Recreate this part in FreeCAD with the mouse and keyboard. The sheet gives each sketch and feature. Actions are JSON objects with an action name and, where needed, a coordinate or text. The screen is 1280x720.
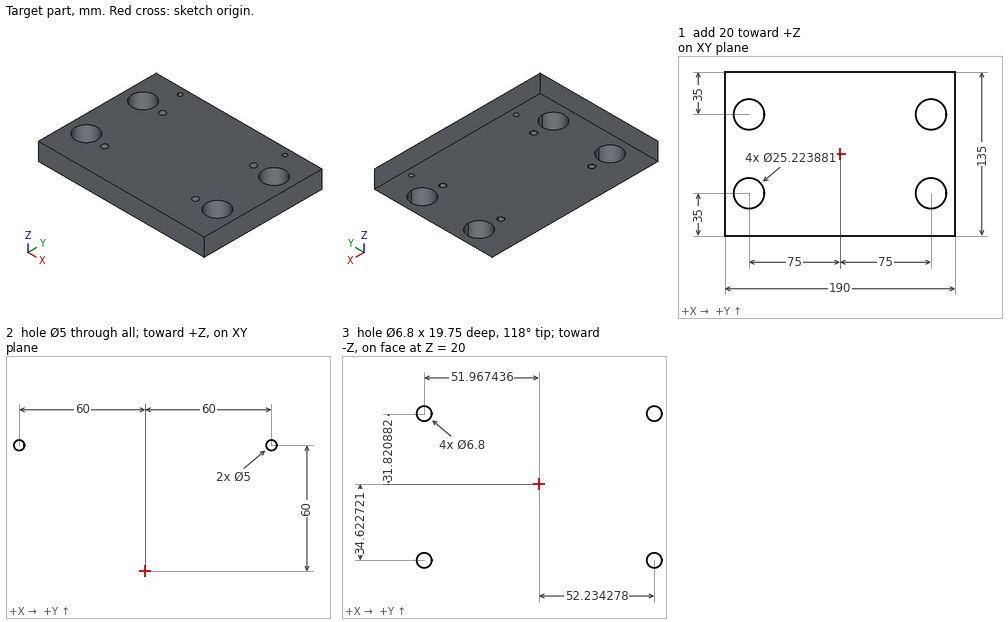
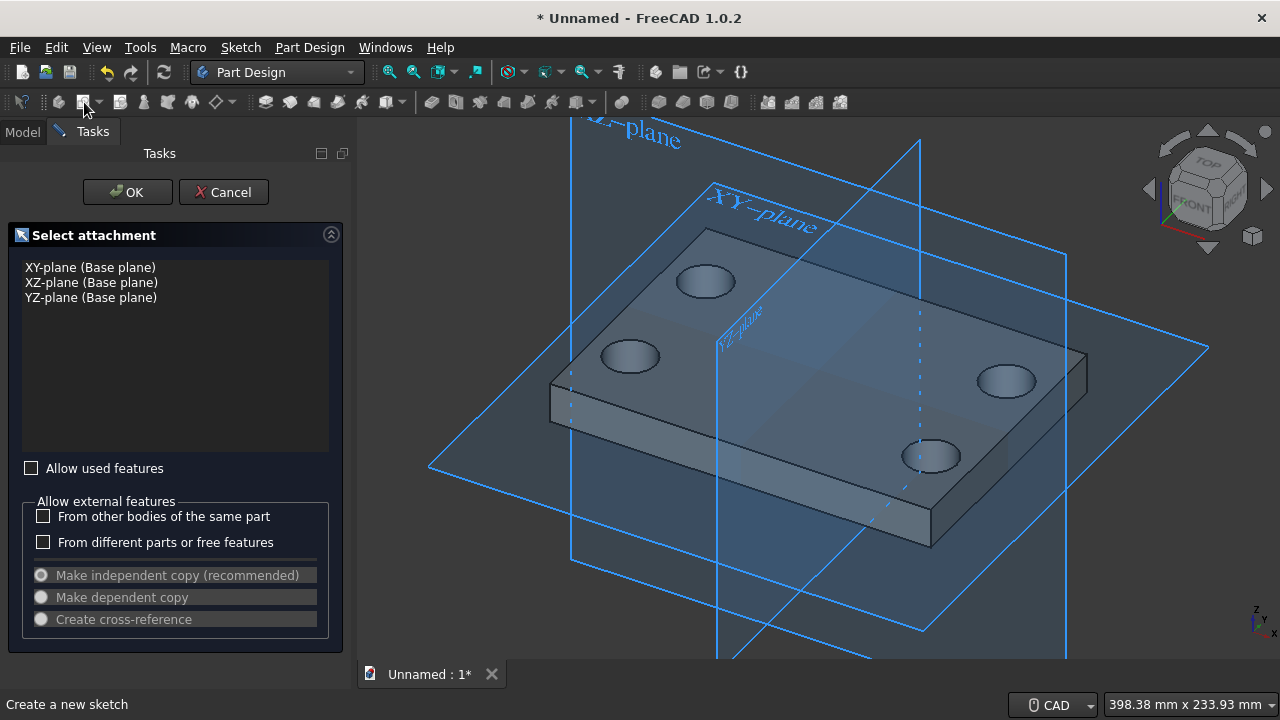
{"action": "left_click", "coordinate": [82, 268]}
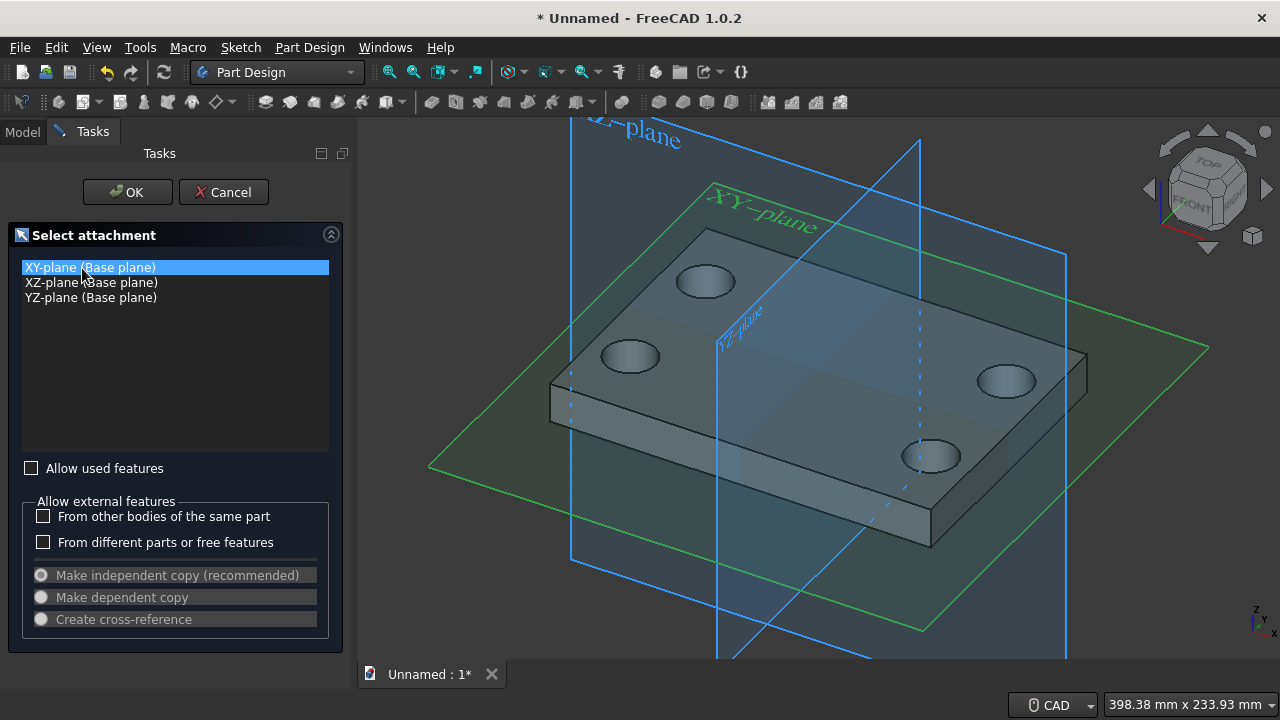
{"action": "left_click", "coordinate": [128, 192]}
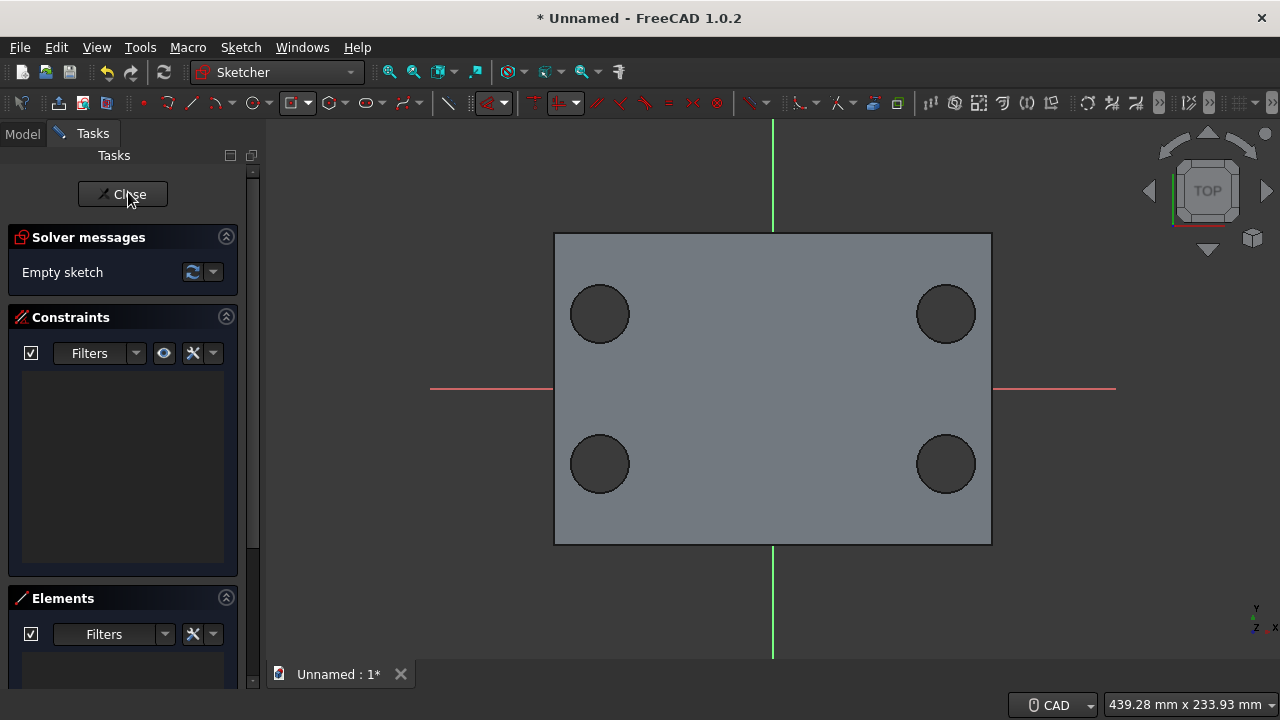
{"action": "left_click", "coordinate": [108, 104]}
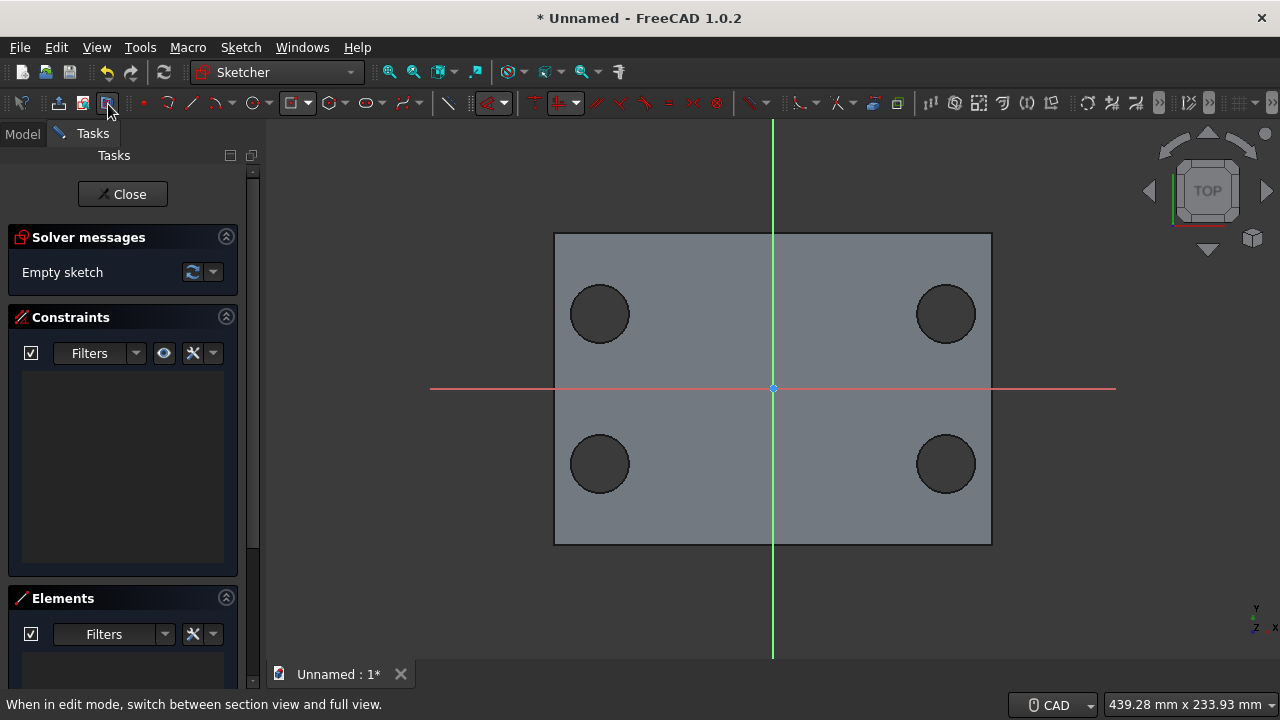
{"action": "scroll", "coordinate": [856, 229], "scroll_direction": "up", "scroll_amount": 3}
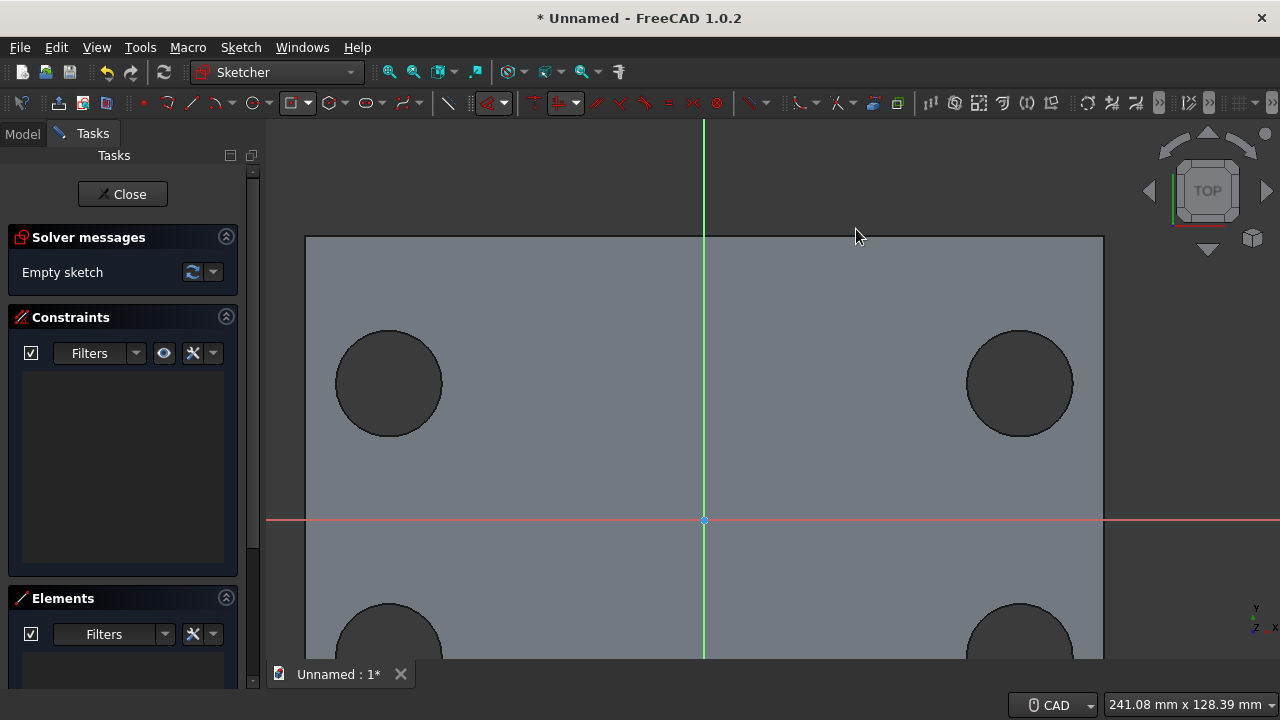
{"action": "key", "text": "g c"}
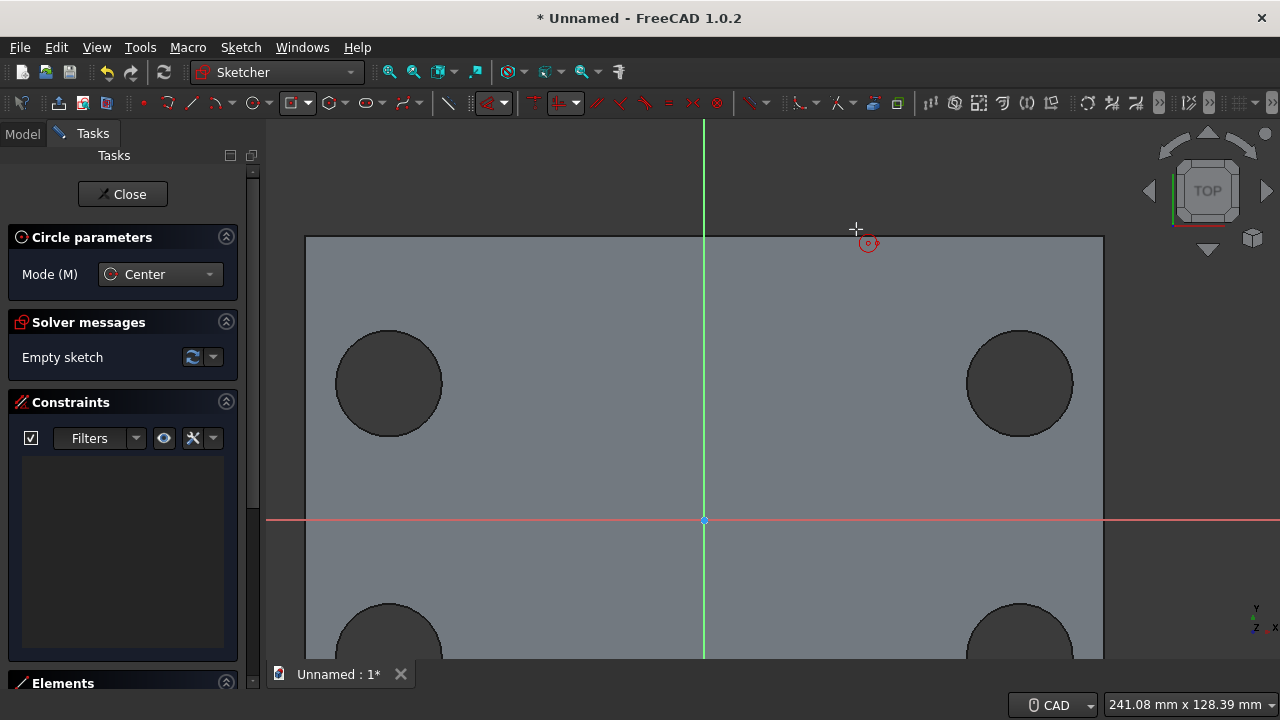
{"action": "scroll", "coordinate": [957, 268], "scroll_direction": "up", "scroll_amount": 4}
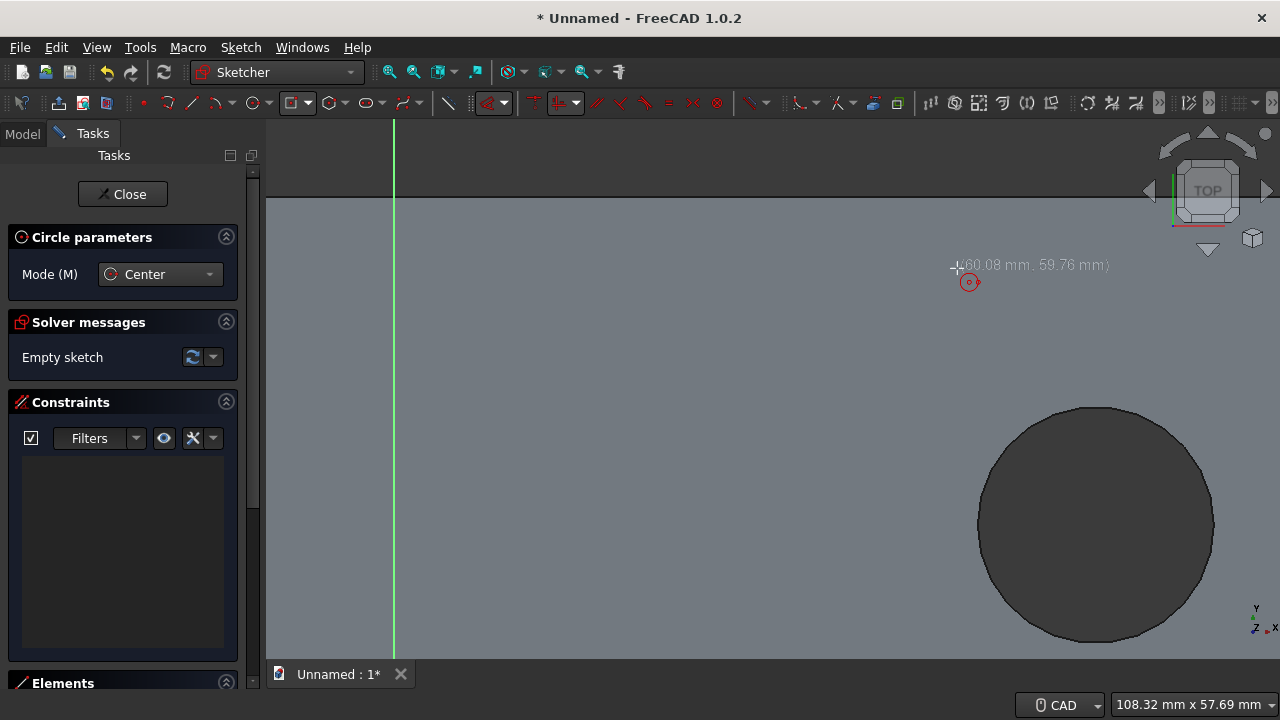
{"action": "left_click", "coordinate": [955, 268]}
{"action": "mouse_move", "coordinate": [972, 251]}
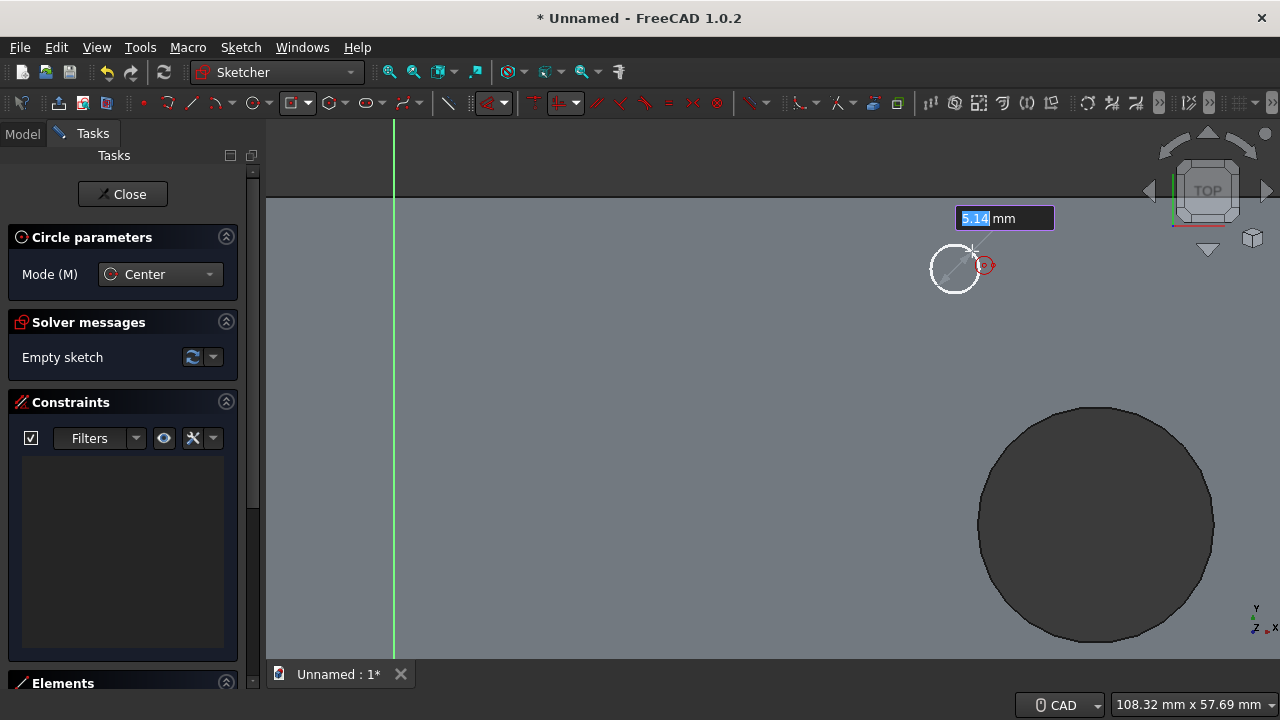
{"action": "type", "text": "5"}
{"action": "key", "text": "Return"}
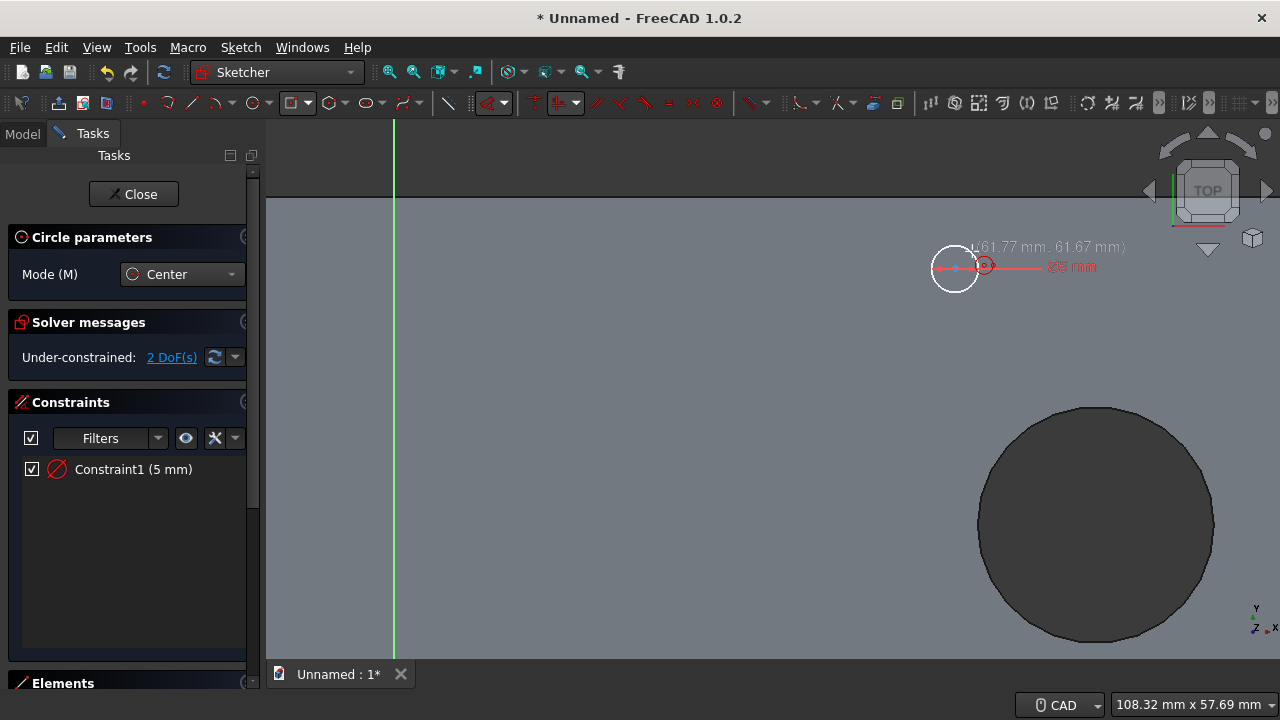
{"action": "scroll", "coordinate": [958, 268], "scroll_direction": "down", "scroll_amount": 4}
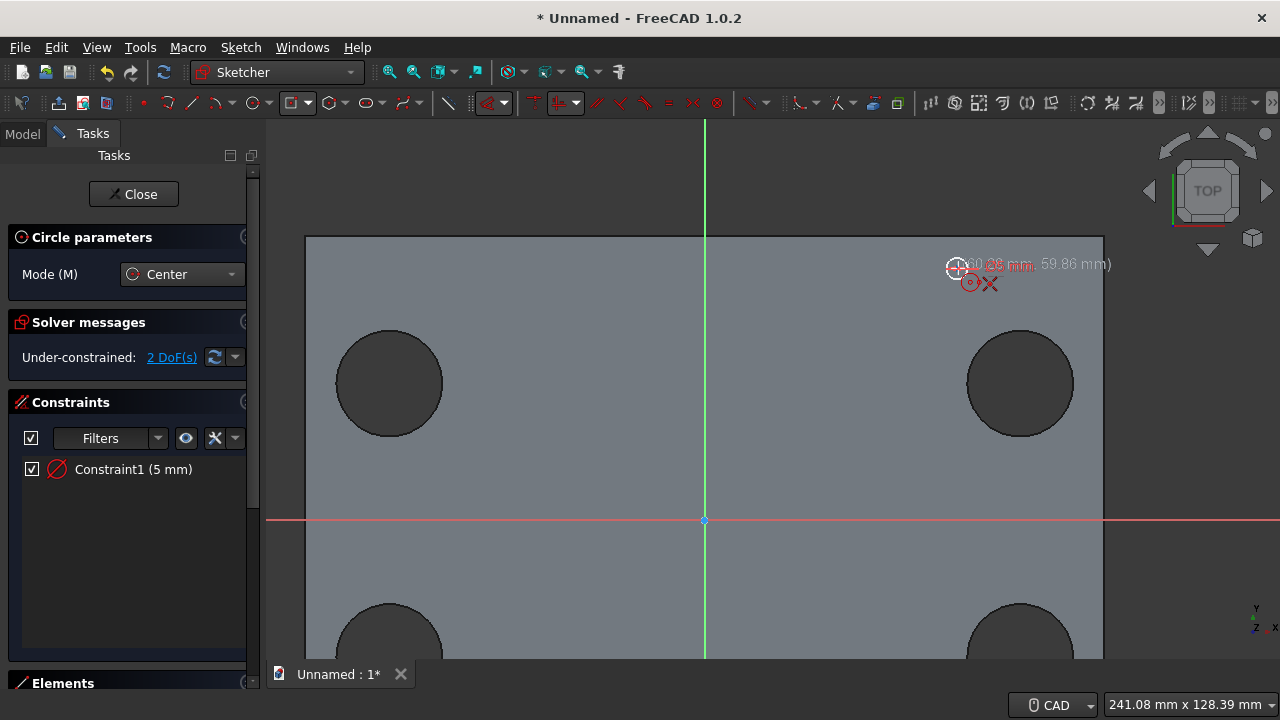
{"action": "scroll", "coordinate": [452, 268], "scroll_direction": "up", "scroll_amount": 4}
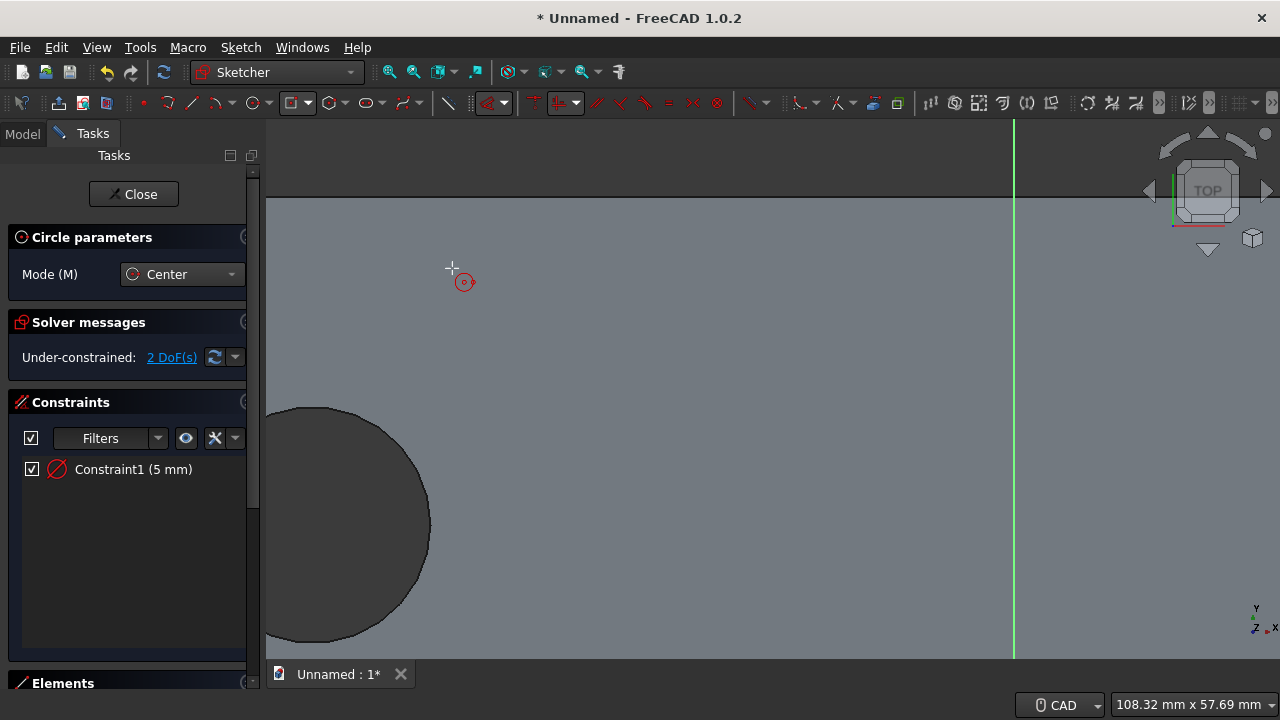
{"action": "left_click", "coordinate": [453, 268]}
{"action": "mouse_move", "coordinate": [469, 251]}